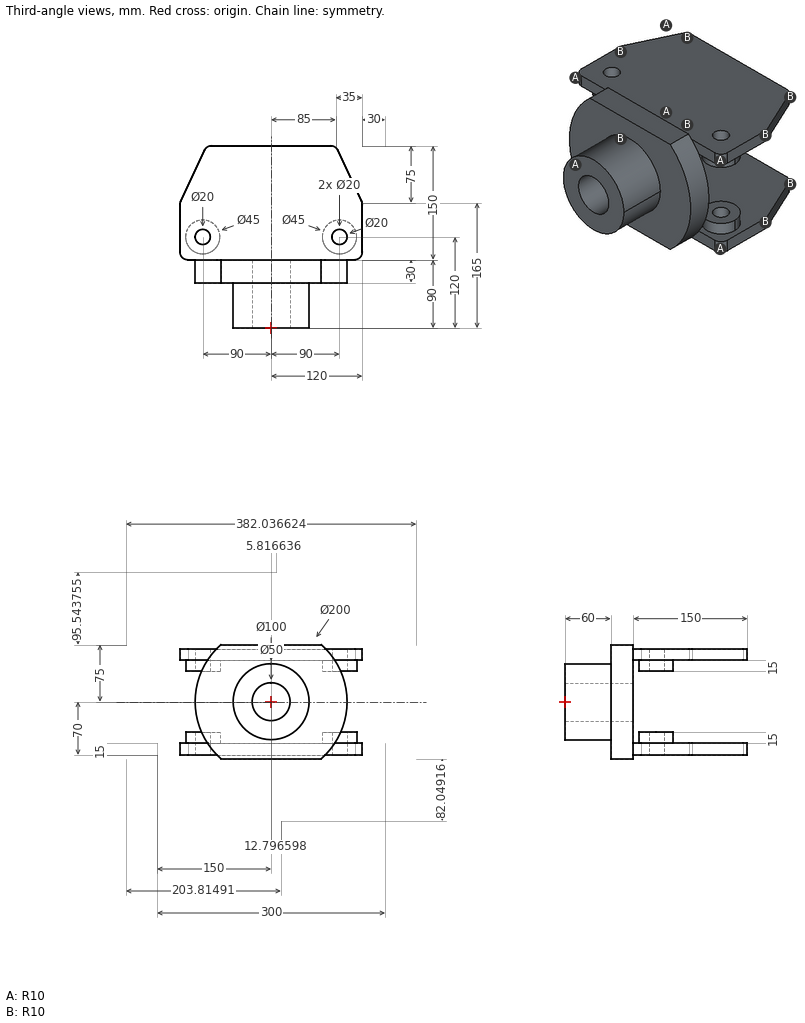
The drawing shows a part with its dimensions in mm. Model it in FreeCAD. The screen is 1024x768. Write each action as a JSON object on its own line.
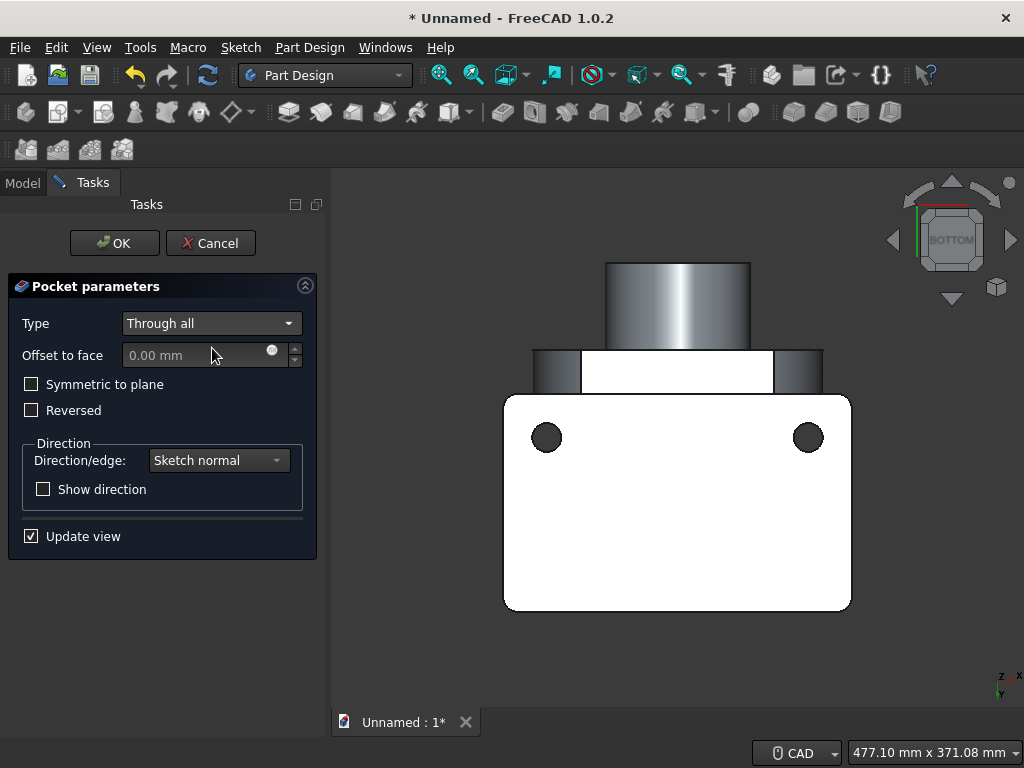
{"action": "left_click", "coordinate": [115, 243]}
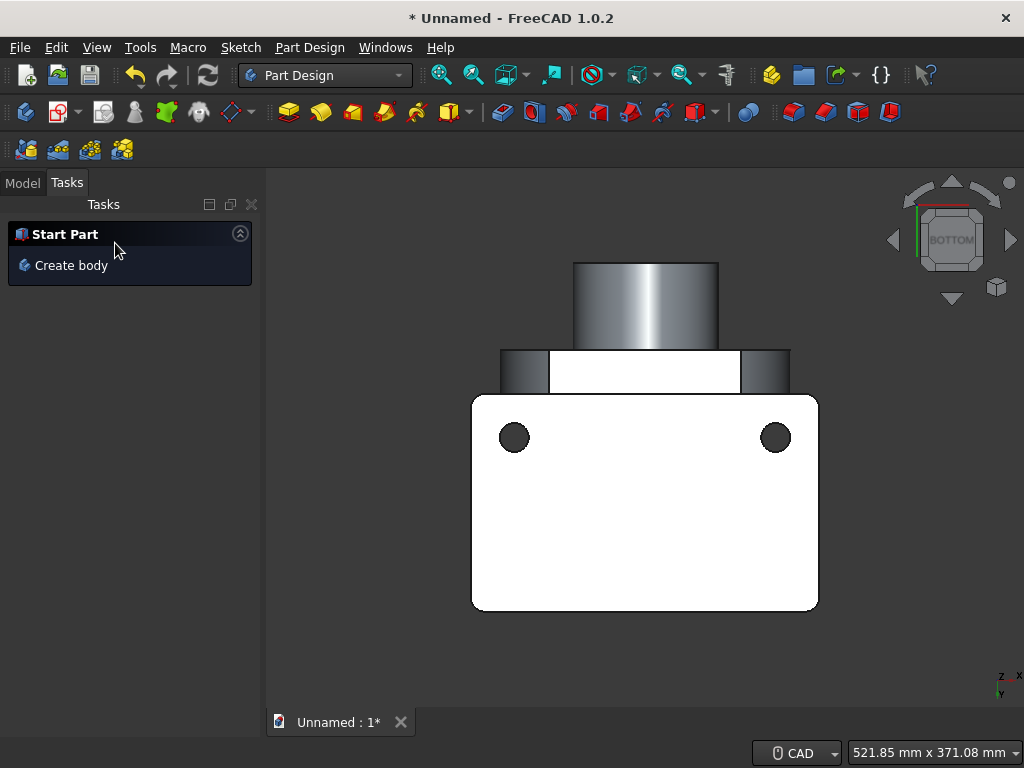
{"action": "left_click", "coordinate": [645, 502]}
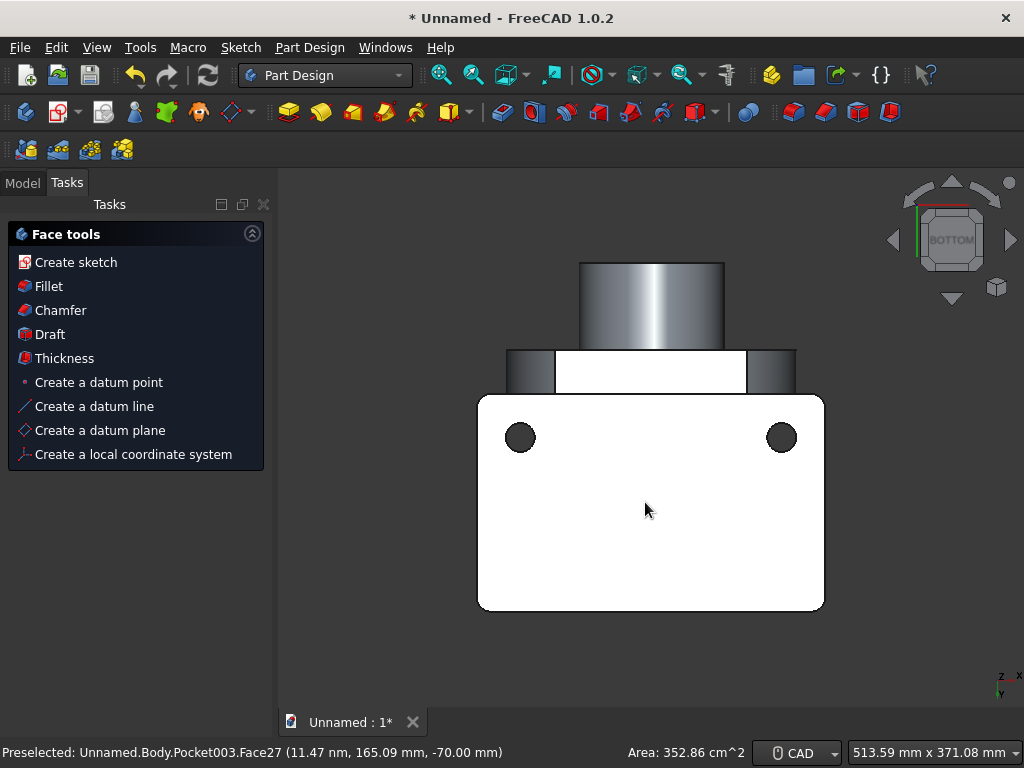
{"action": "left_click", "coordinate": [58, 112]}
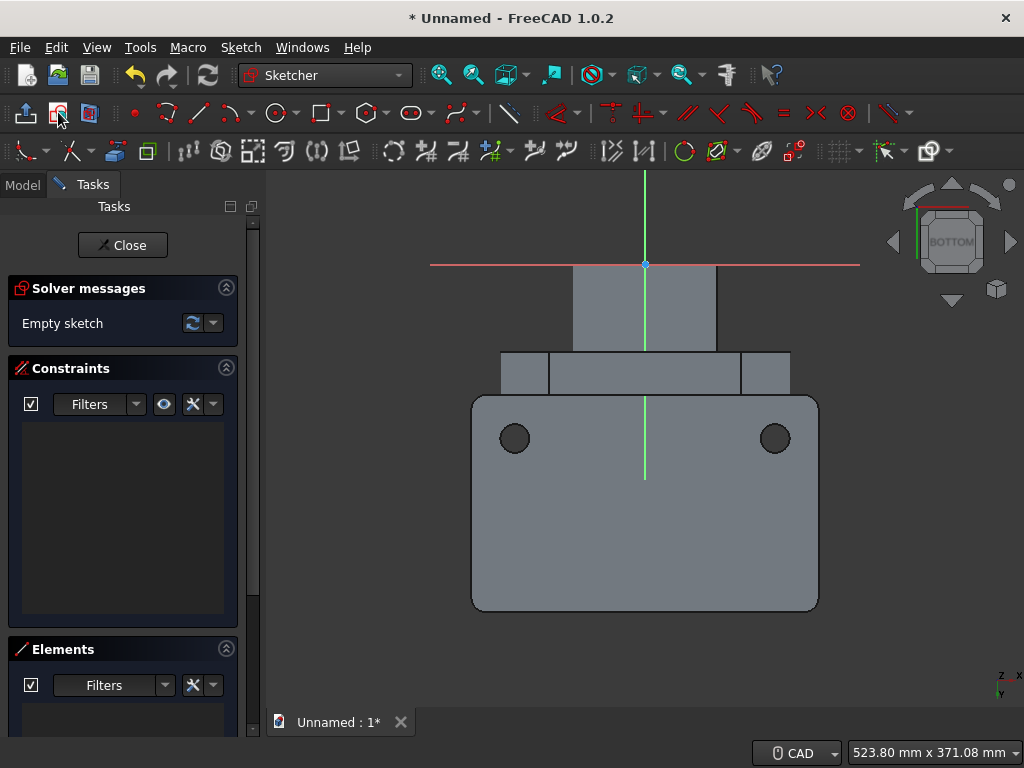
{"action": "key", "text": "q s"}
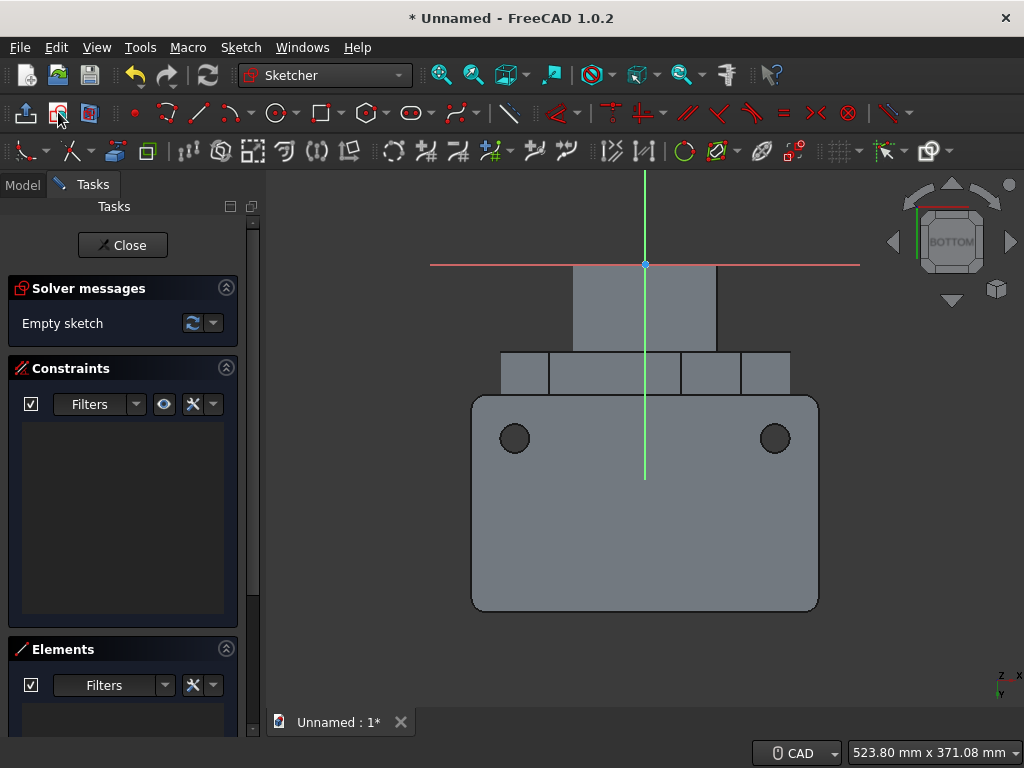
{"action": "left_click", "coordinate": [168, 114]}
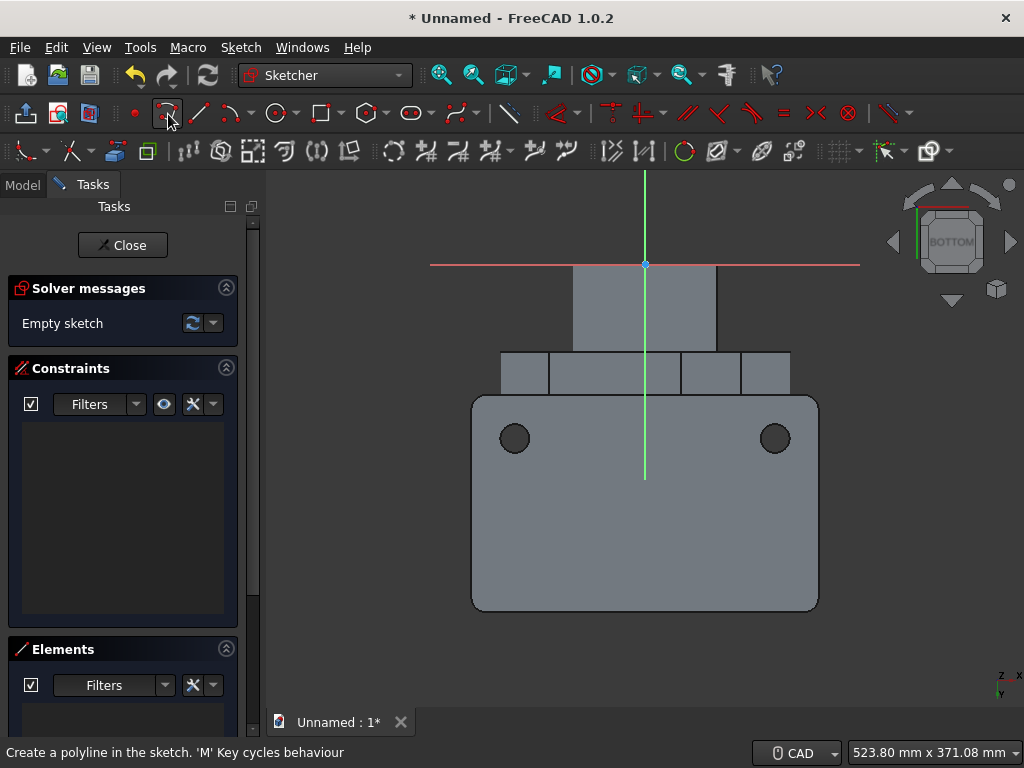
{"action": "left_click", "coordinate": [819, 504]}
{"action": "left_click", "coordinate": [768, 612]}
{"action": "left_click", "coordinate": [819, 612]}
{"action": "left_click", "coordinate": [819, 505]}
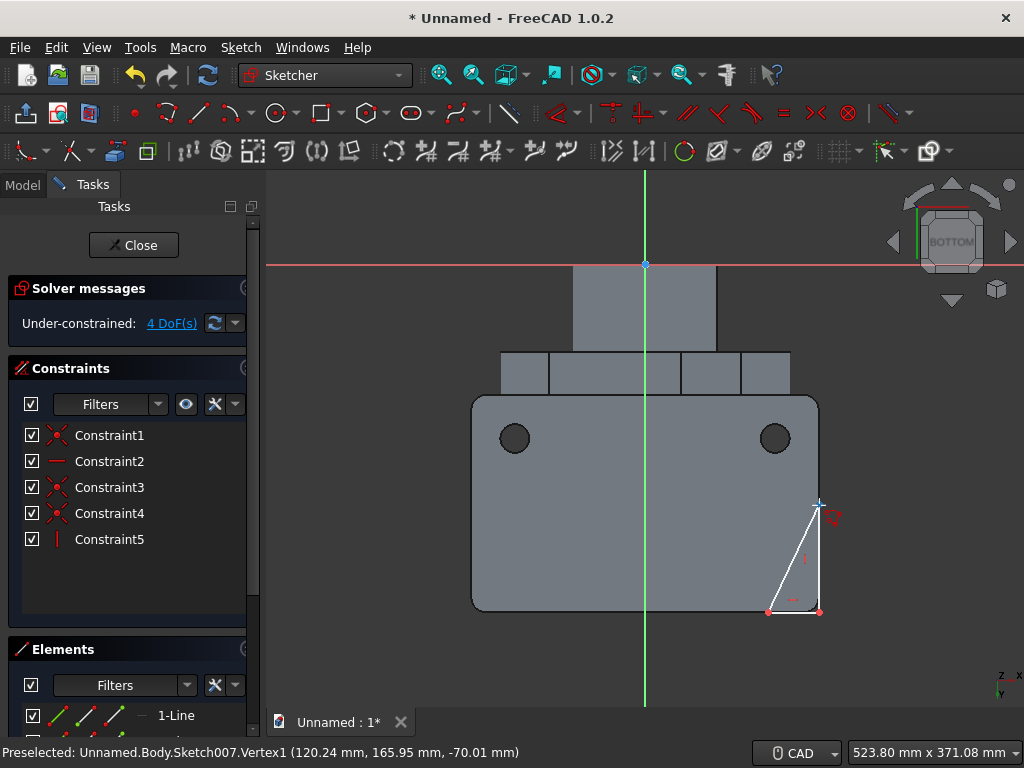
{"action": "left_click", "coordinate": [471, 504]}
{"action": "left_click", "coordinate": [471, 612]}
{"action": "left_click", "coordinate": [522, 612]}
{"action": "left_click", "coordinate": [471, 505]}
{"action": "key", "text": "Escape"}
{"action": "key", "text": "Escape"}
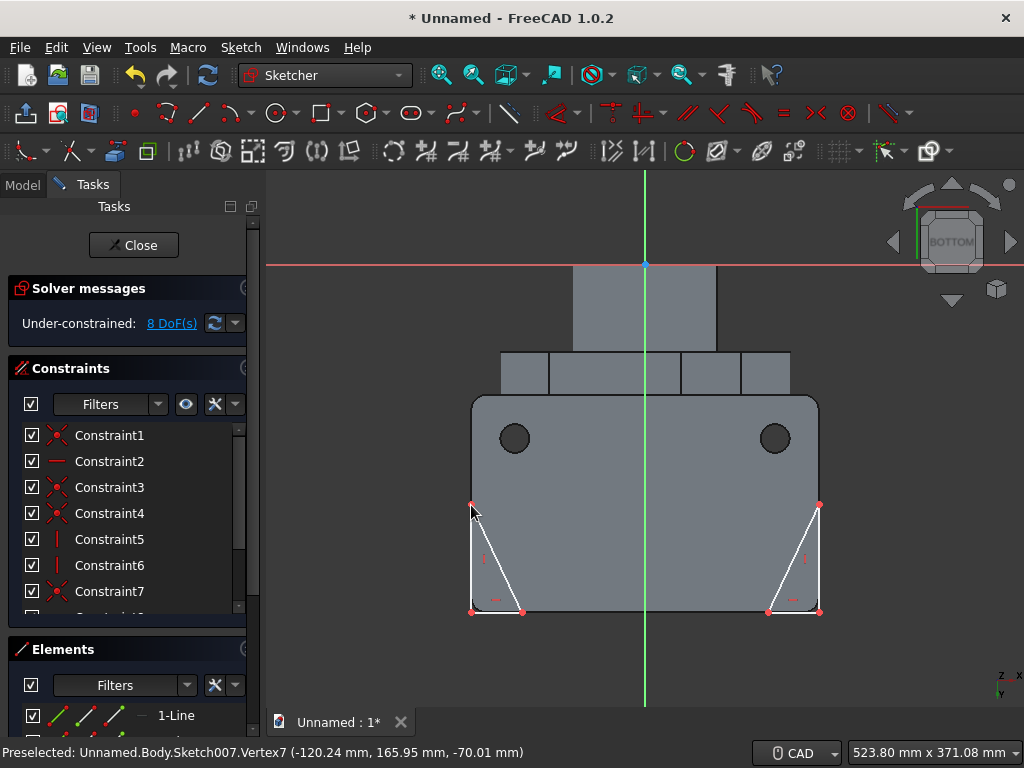
{"action": "left_click", "coordinate": [819, 505]}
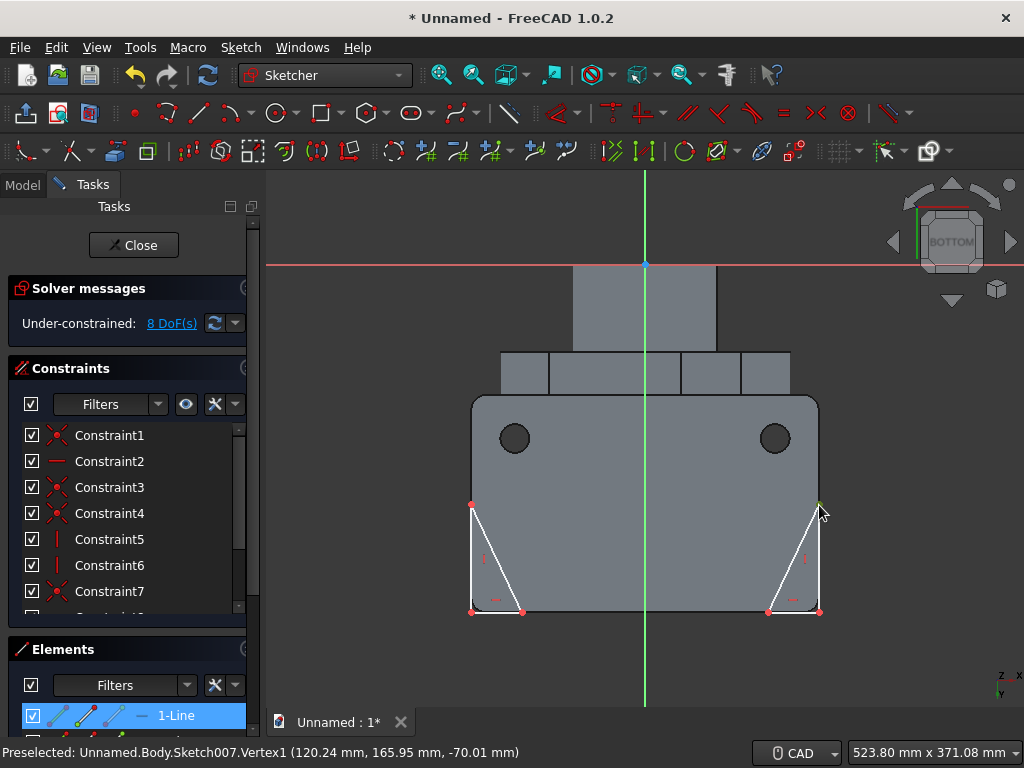
{"action": "left_click", "coordinate": [471, 505]}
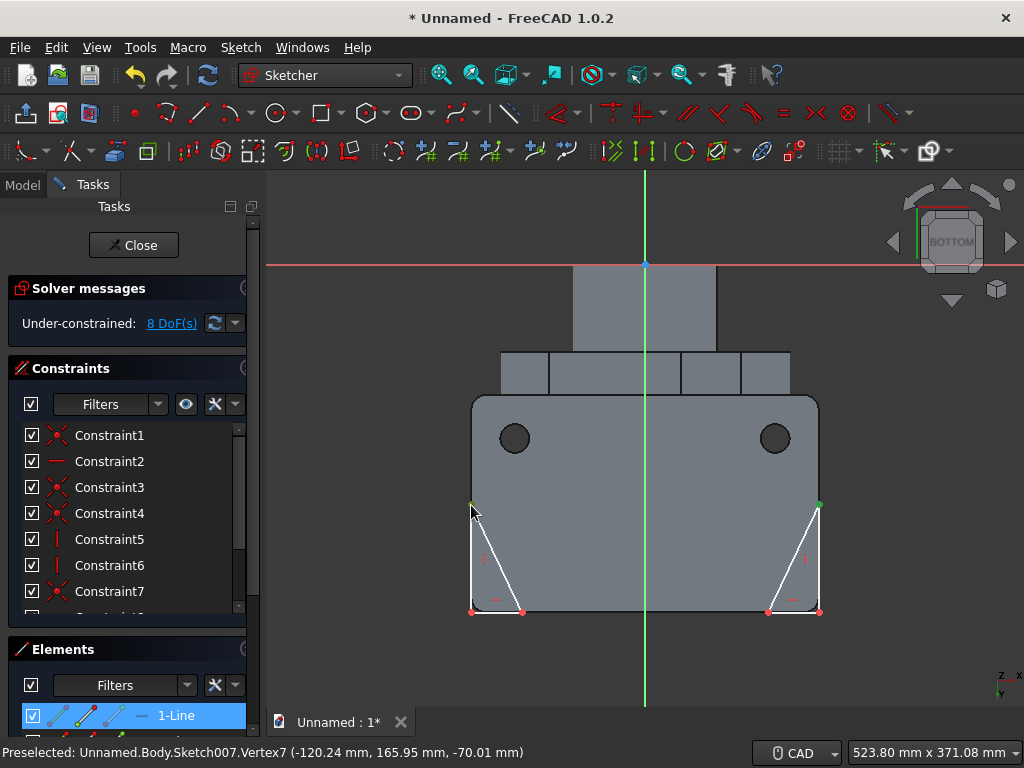
{"action": "left_click", "coordinate": [645, 645]}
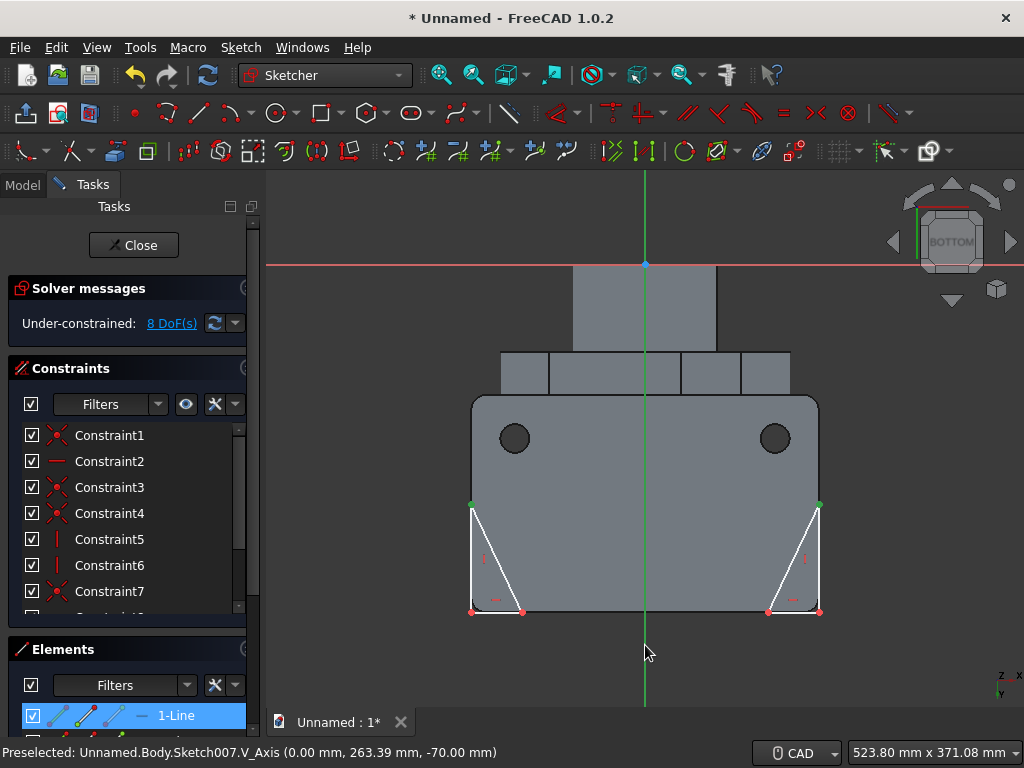
{"action": "left_click", "coordinate": [816, 114]}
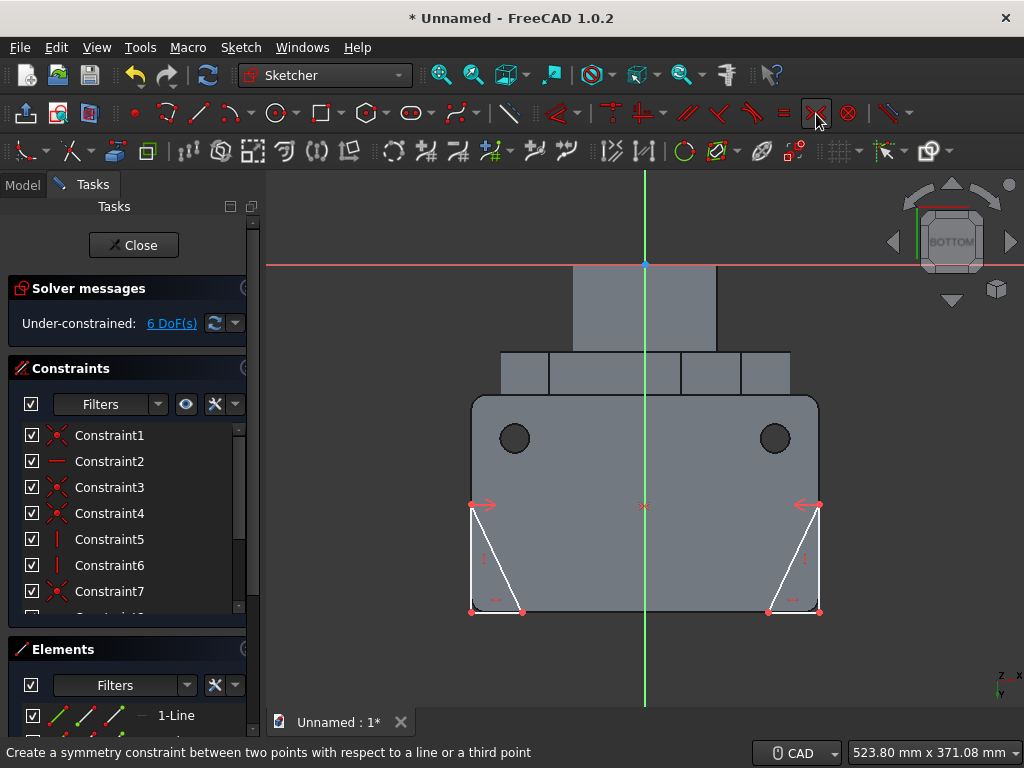
{"action": "left_click", "coordinate": [768, 613]}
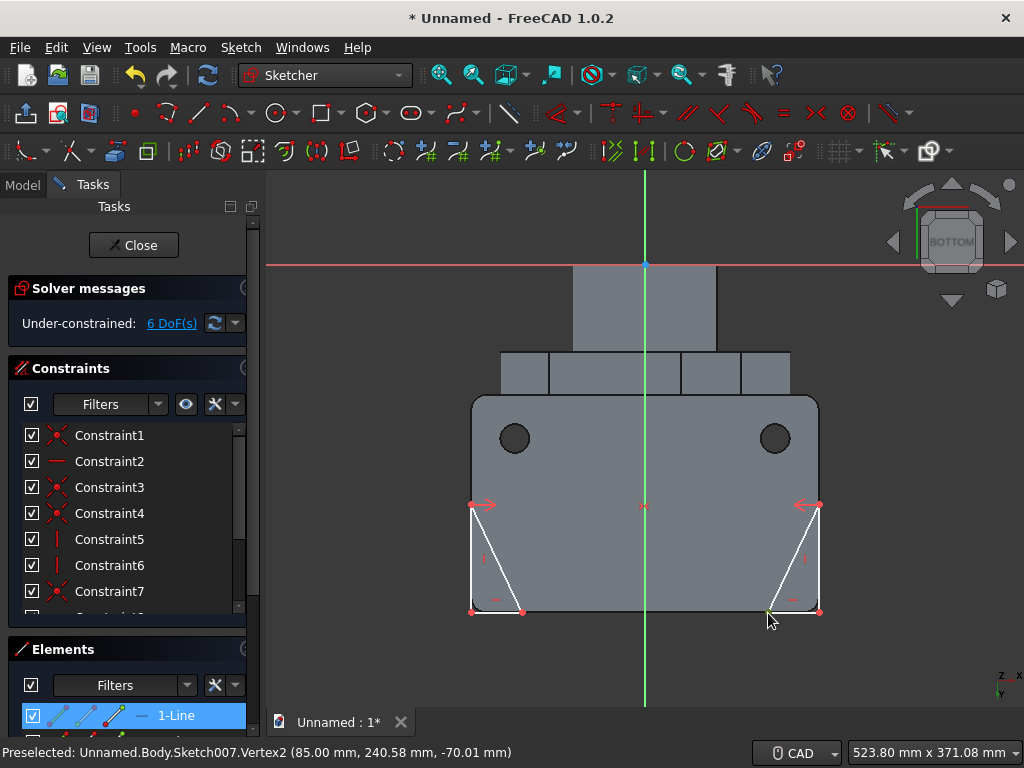
{"action": "left_click", "coordinate": [522, 613]}